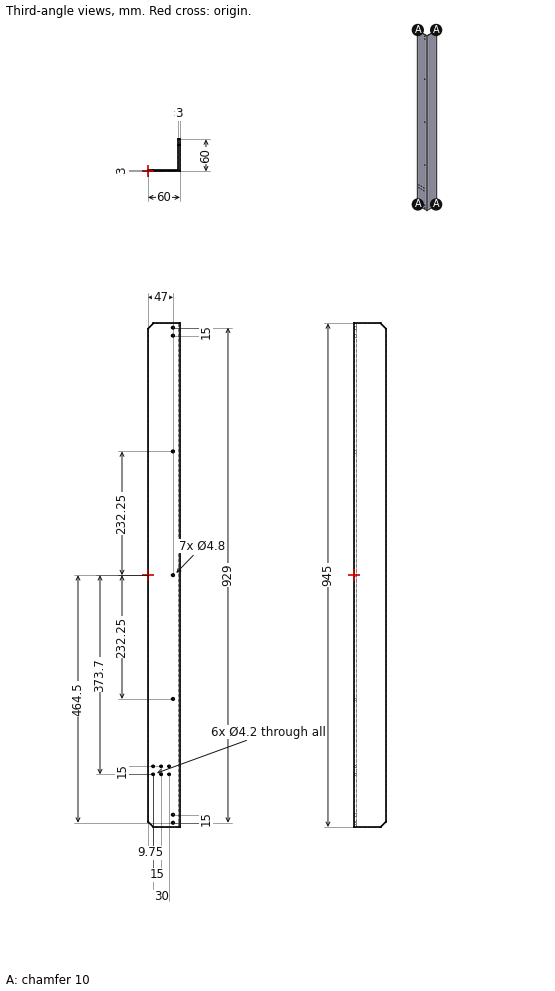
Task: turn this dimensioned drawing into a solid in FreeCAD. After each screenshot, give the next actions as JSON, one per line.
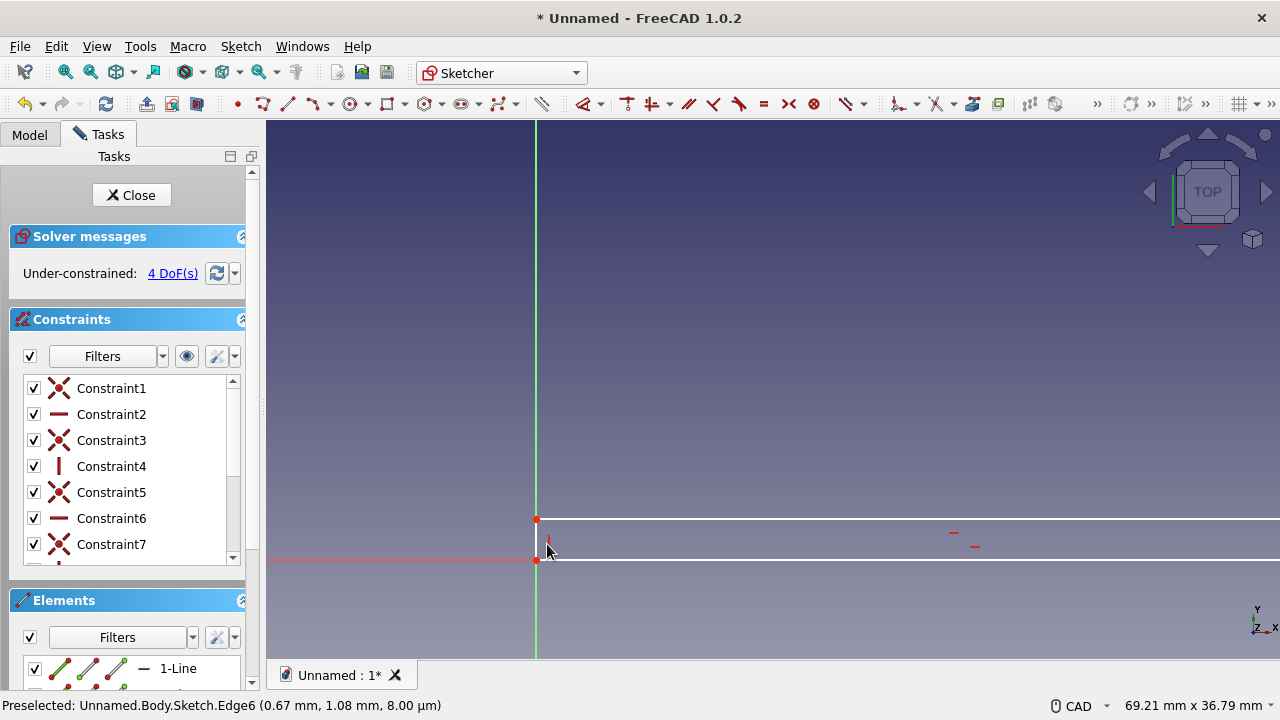
{"action": "left_click", "coordinate": [582, 104]}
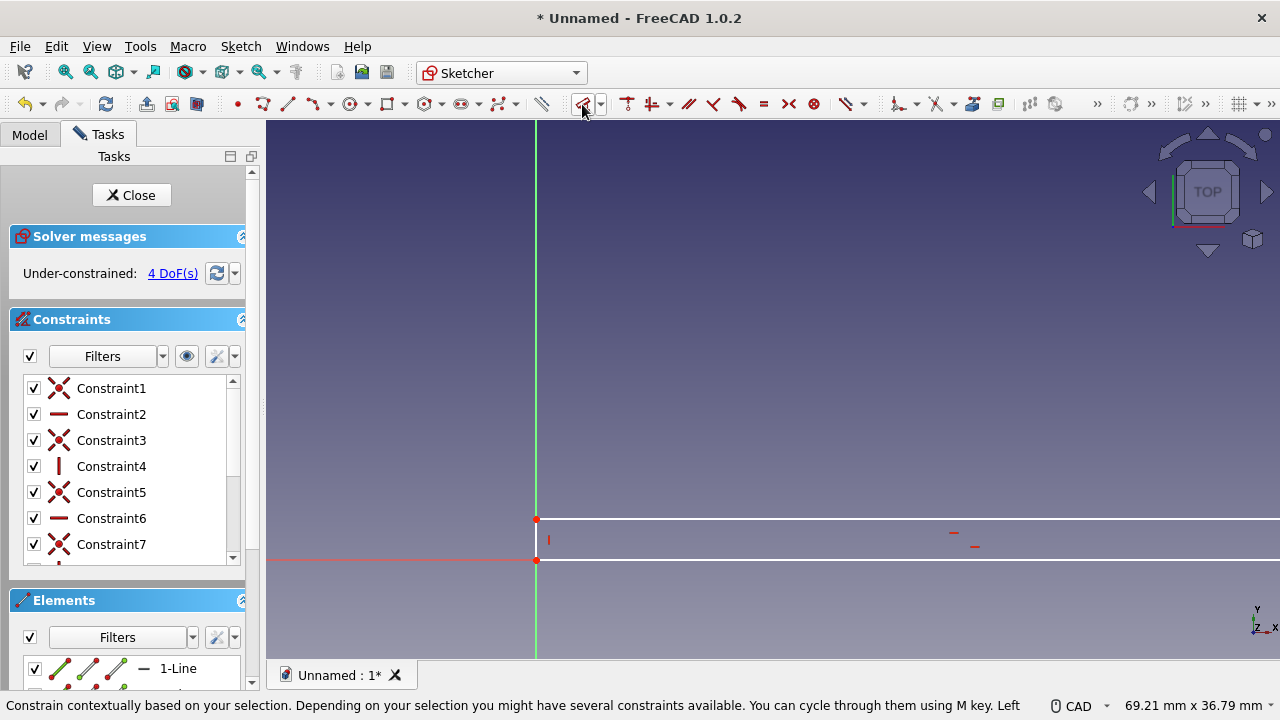
{"action": "scroll", "coordinate": [547, 546], "scroll_direction": "down", "scroll_amount": 5}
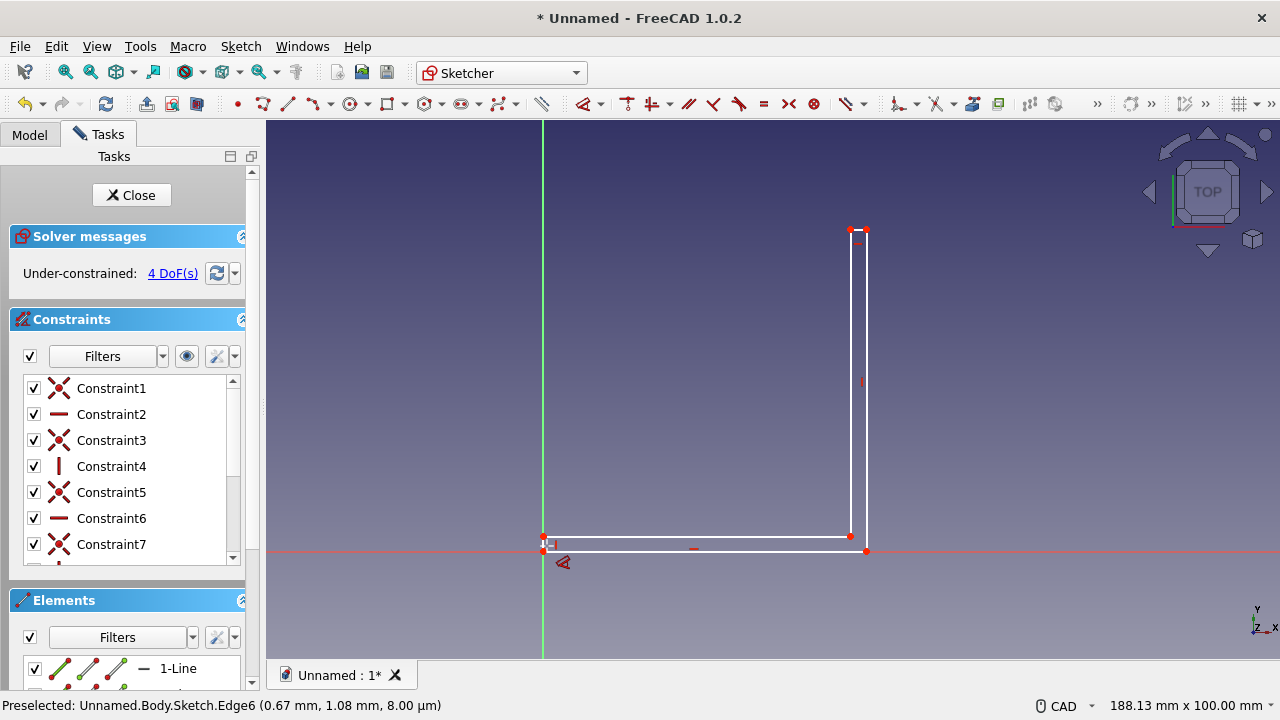
{"action": "scroll", "coordinate": [862, 230], "scroll_direction": "up", "scroll_amount": 6}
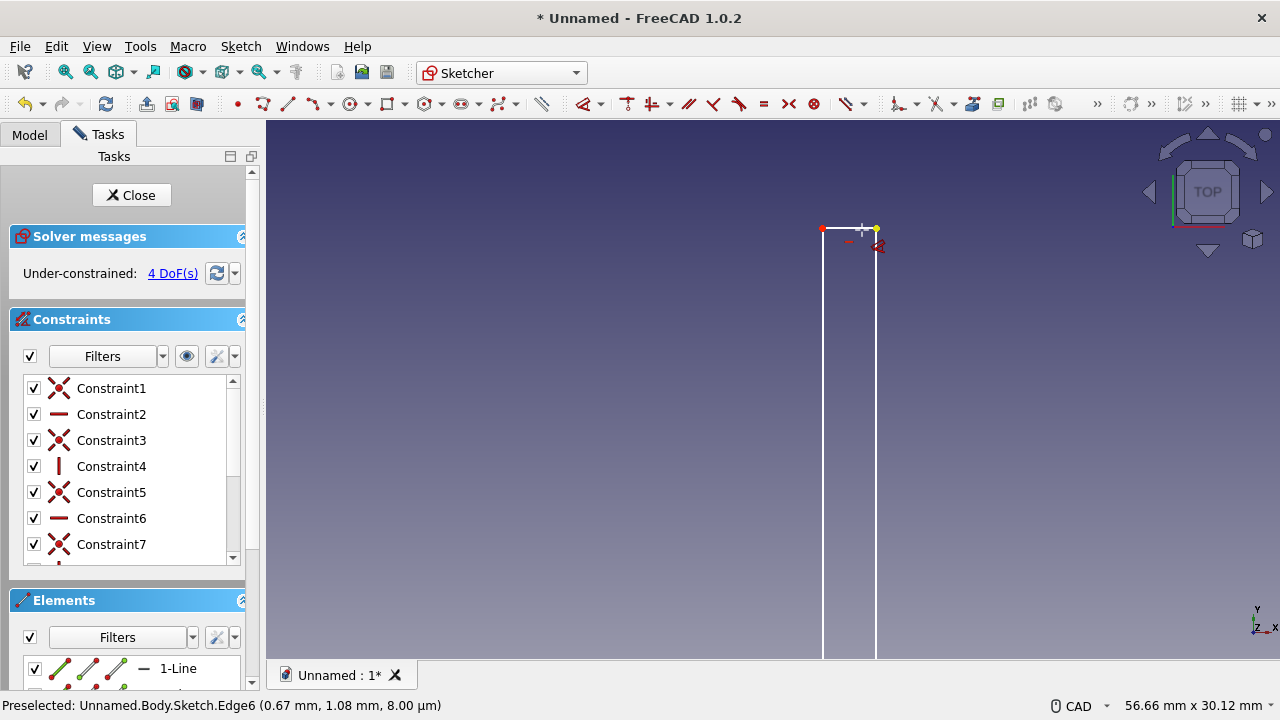
{"action": "left_click", "coordinate": [860, 228]}
{"action": "left_click", "coordinate": [849, 194]}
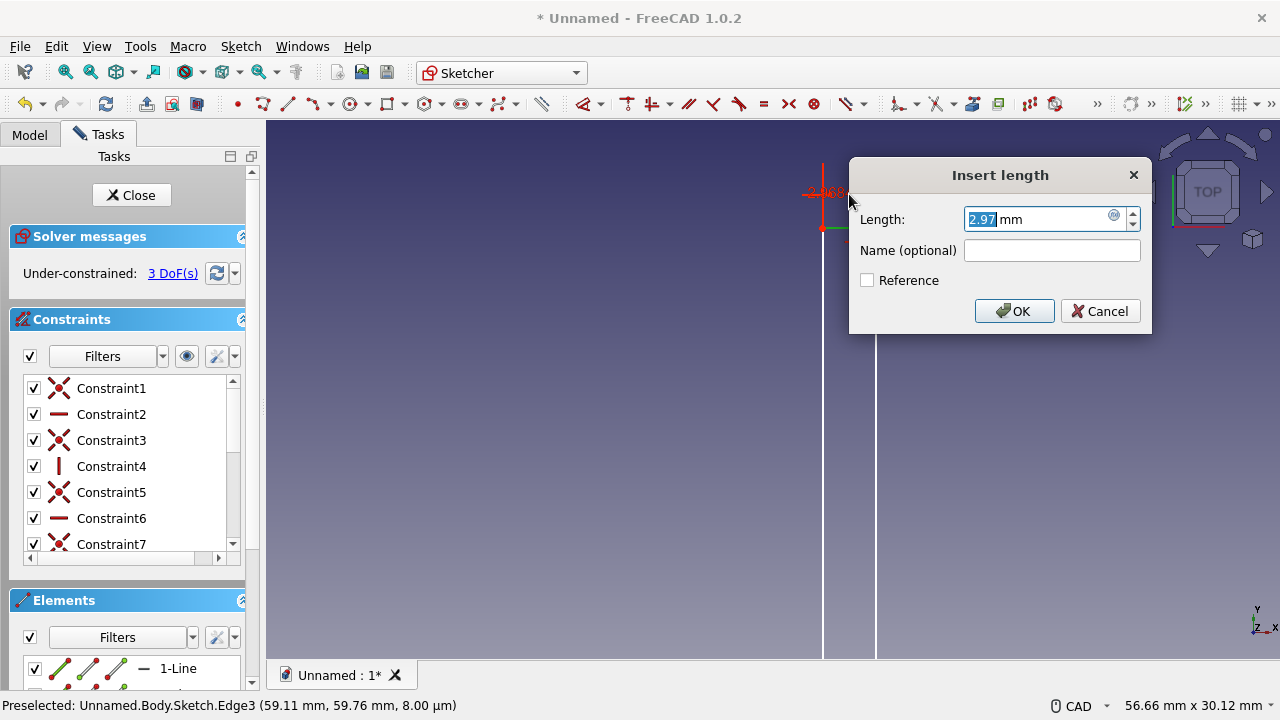
{"action": "type", "text": "3"}
{"action": "key", "text": "Return"}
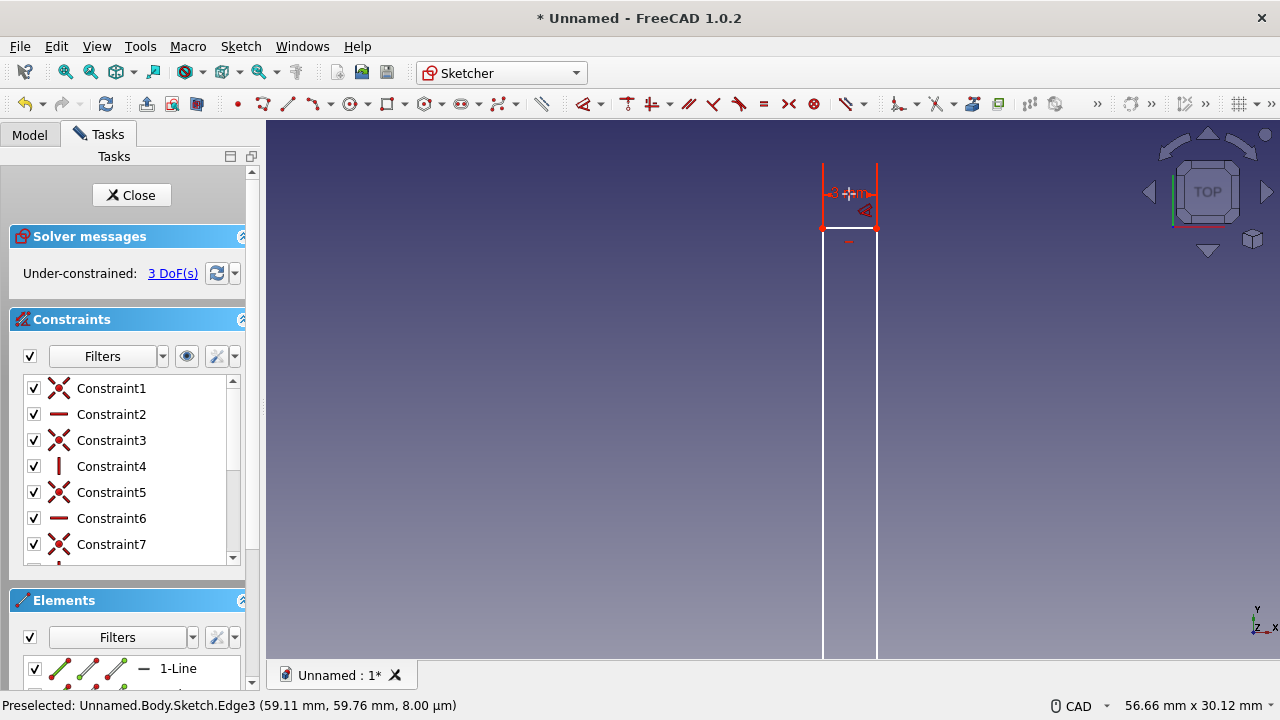
{"action": "scroll", "coordinate": [862, 229], "scroll_direction": "down", "scroll_amount": 6}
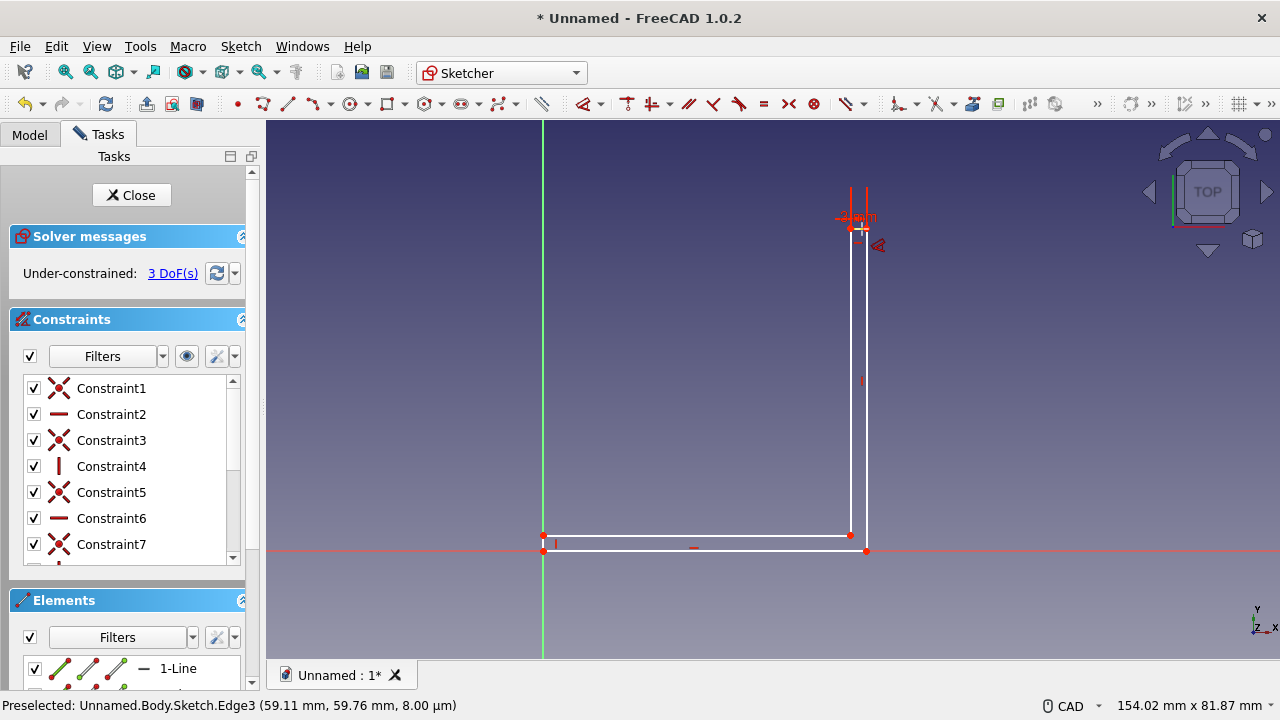
{"action": "scroll", "coordinate": [543, 540], "scroll_direction": "up", "scroll_amount": 6}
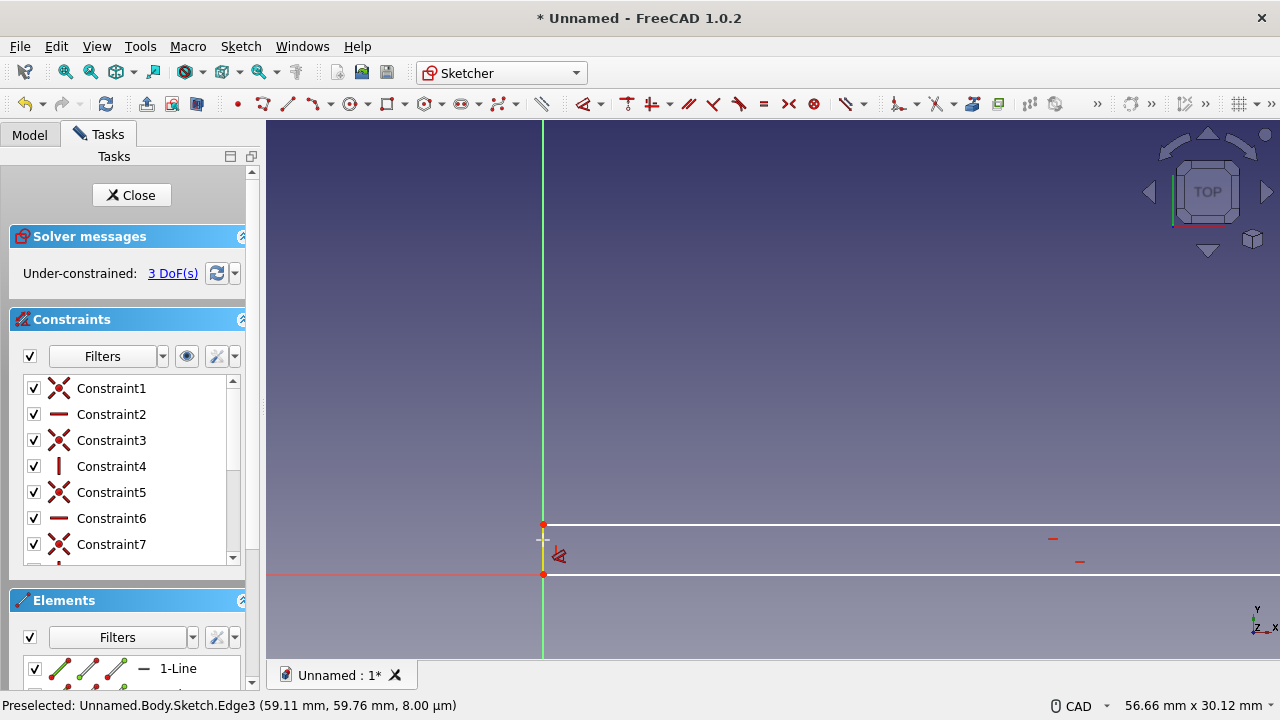
{"action": "left_click", "coordinate": [543, 540]}
{"action": "left_click", "coordinate": [509, 550]}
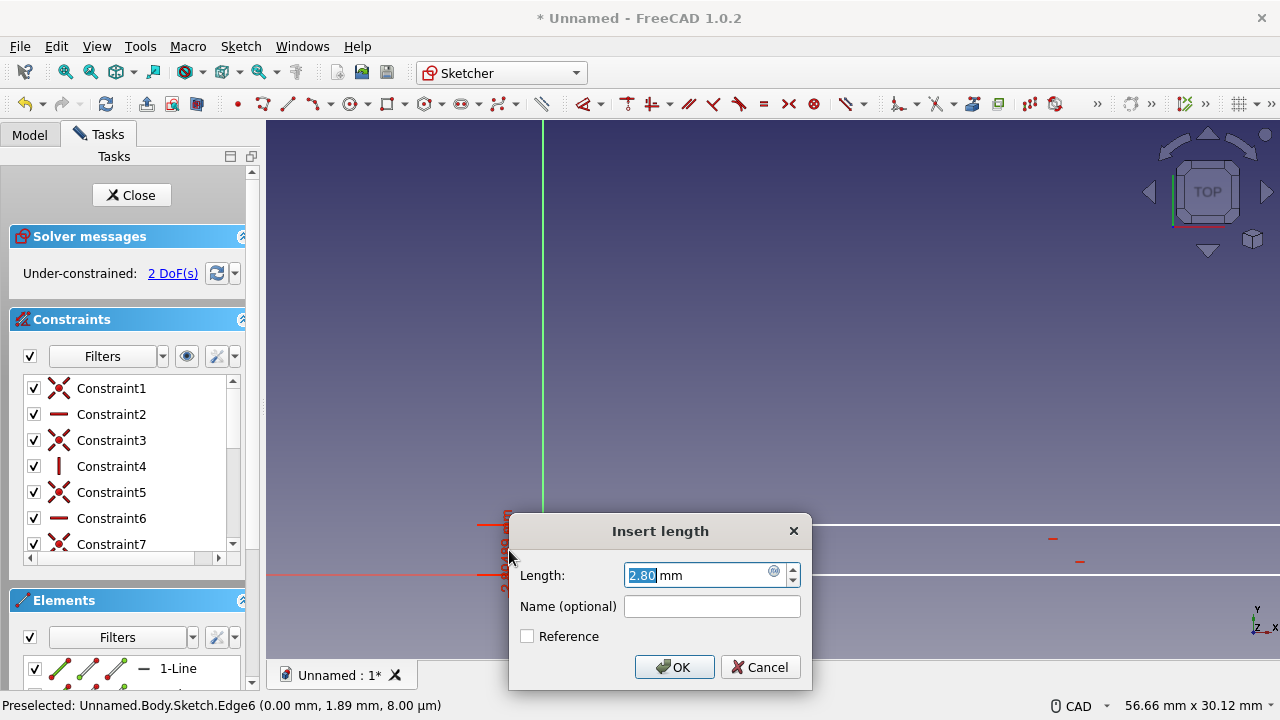
{"action": "type", "text": "3"}
{"action": "key", "text": "Return"}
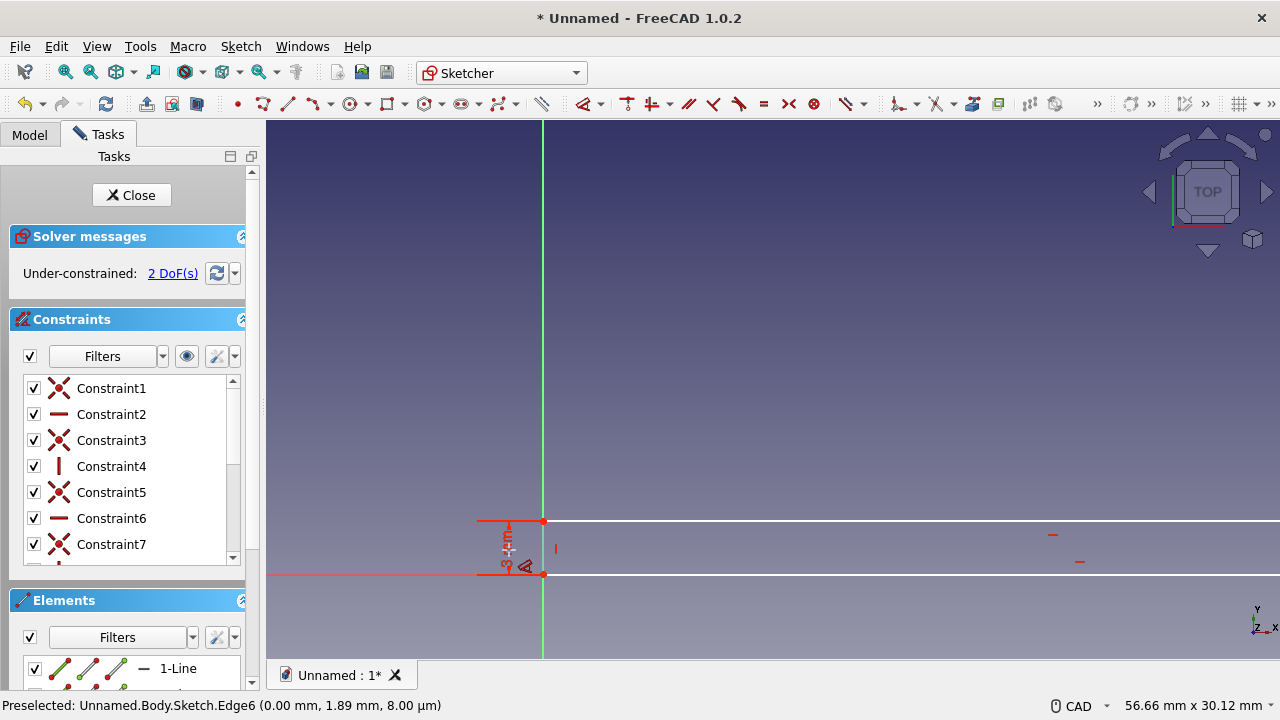
{"action": "left_click", "coordinate": [865, 575]}
{"action": "left_click", "coordinate": [829, 609]}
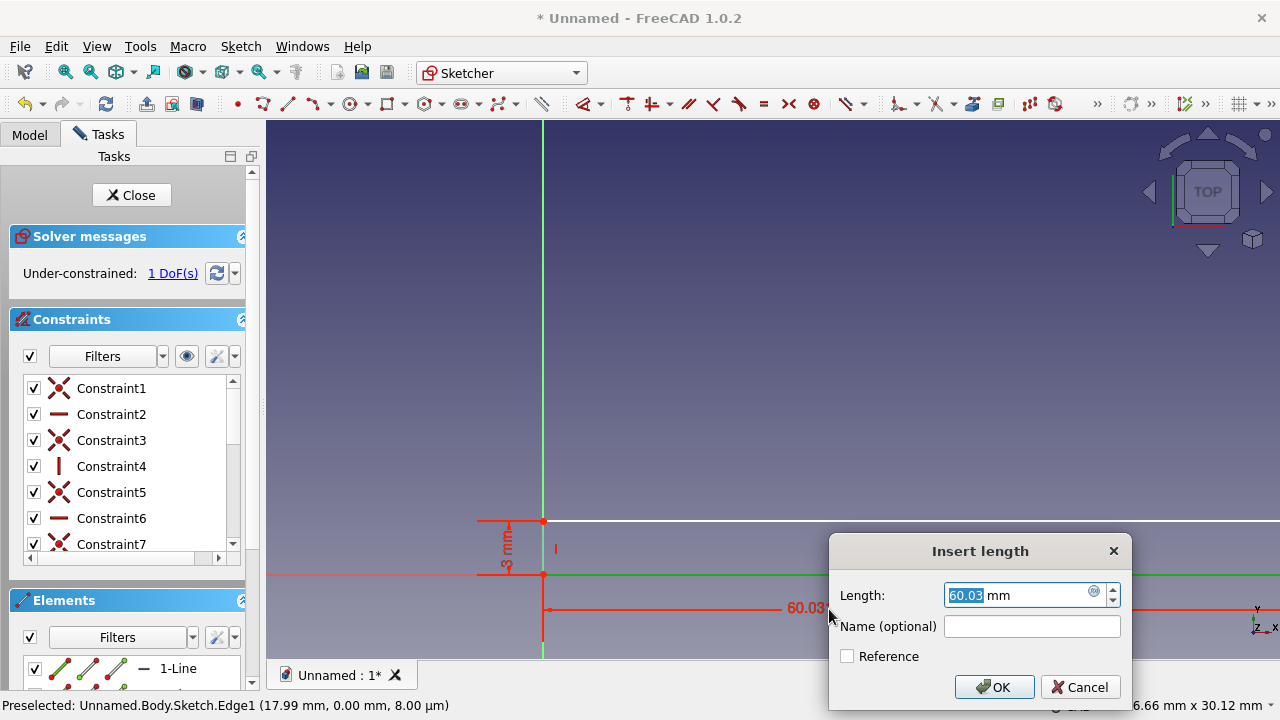
{"action": "type", "text": "60"}
{"action": "key", "text": "Return"}